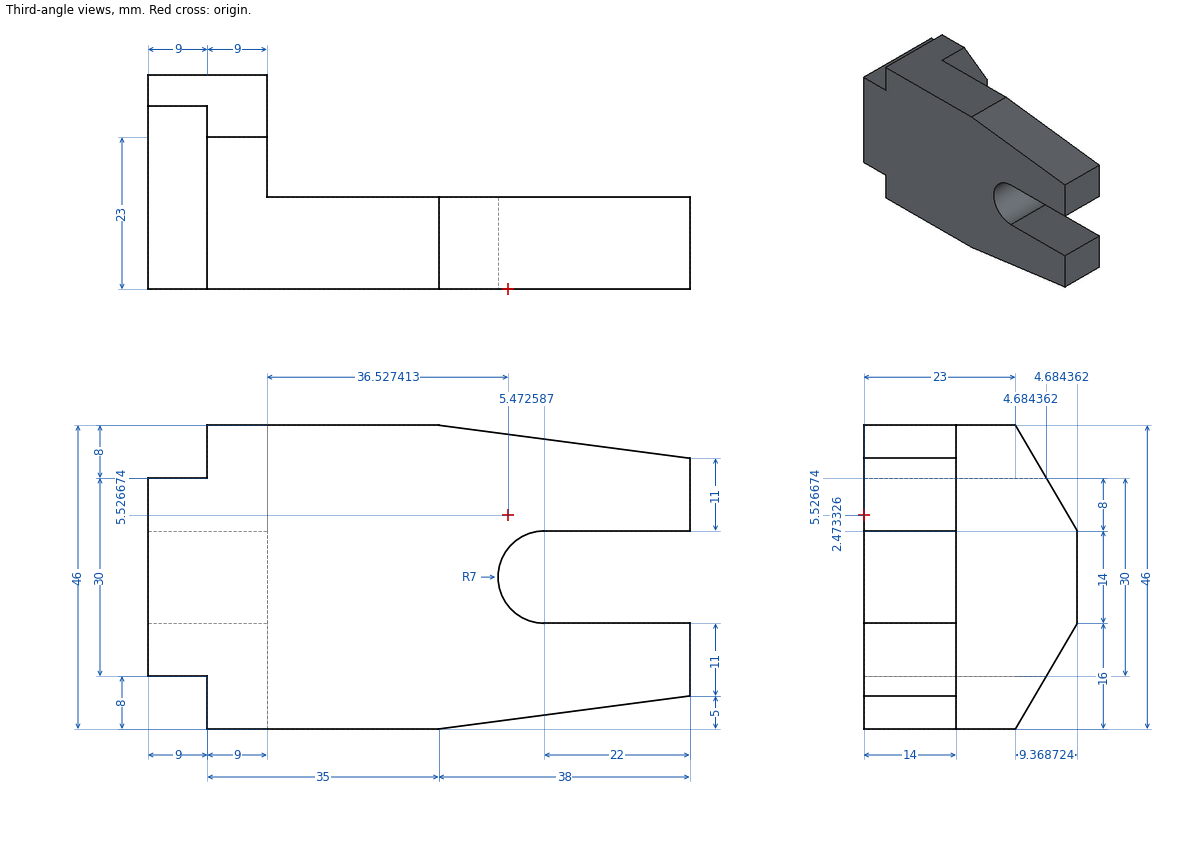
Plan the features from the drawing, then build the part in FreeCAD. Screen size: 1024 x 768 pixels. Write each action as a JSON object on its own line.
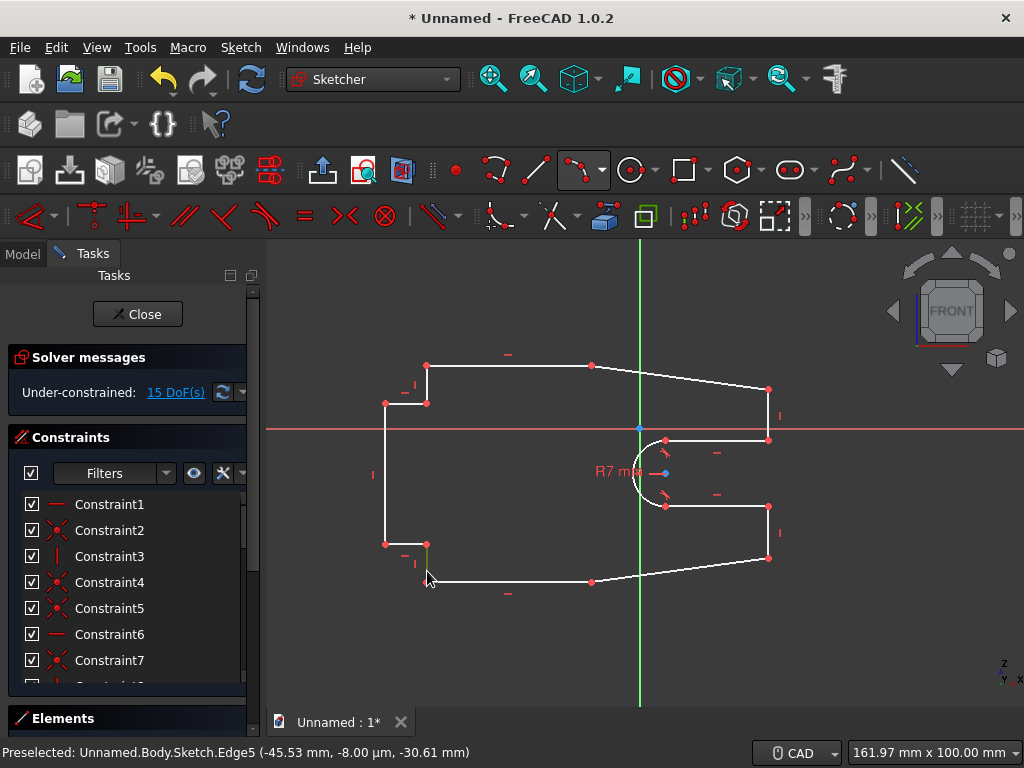
{"action": "left_click", "coordinate": [56, 216]}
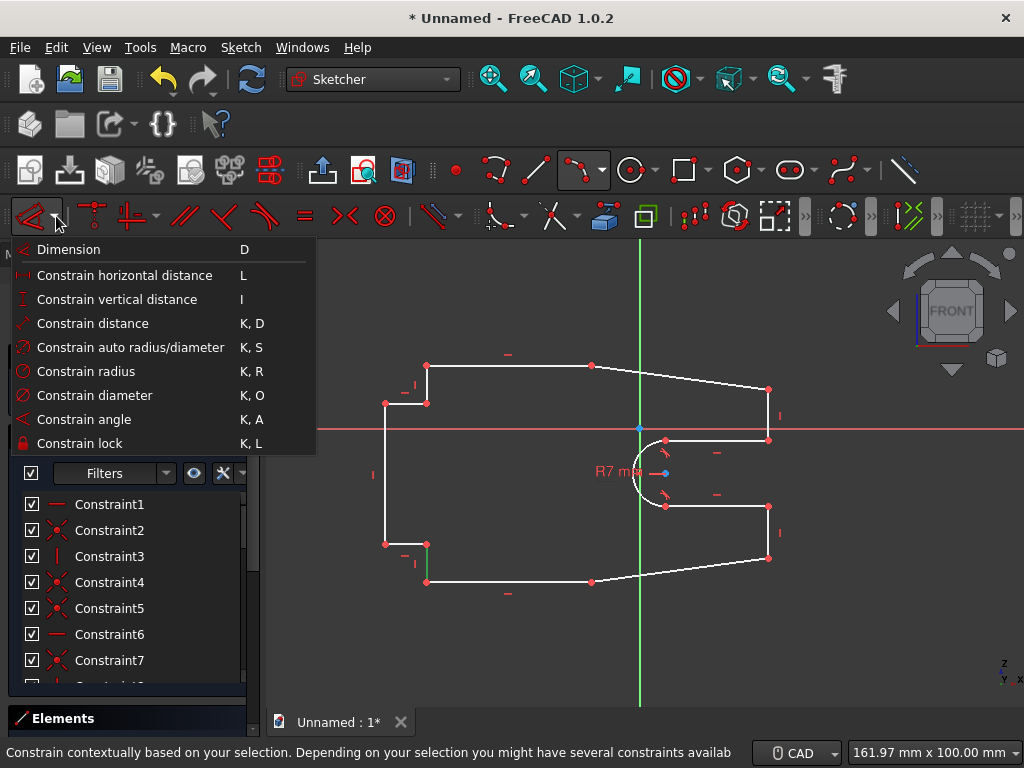
{"action": "left_click", "coordinate": [164, 299]}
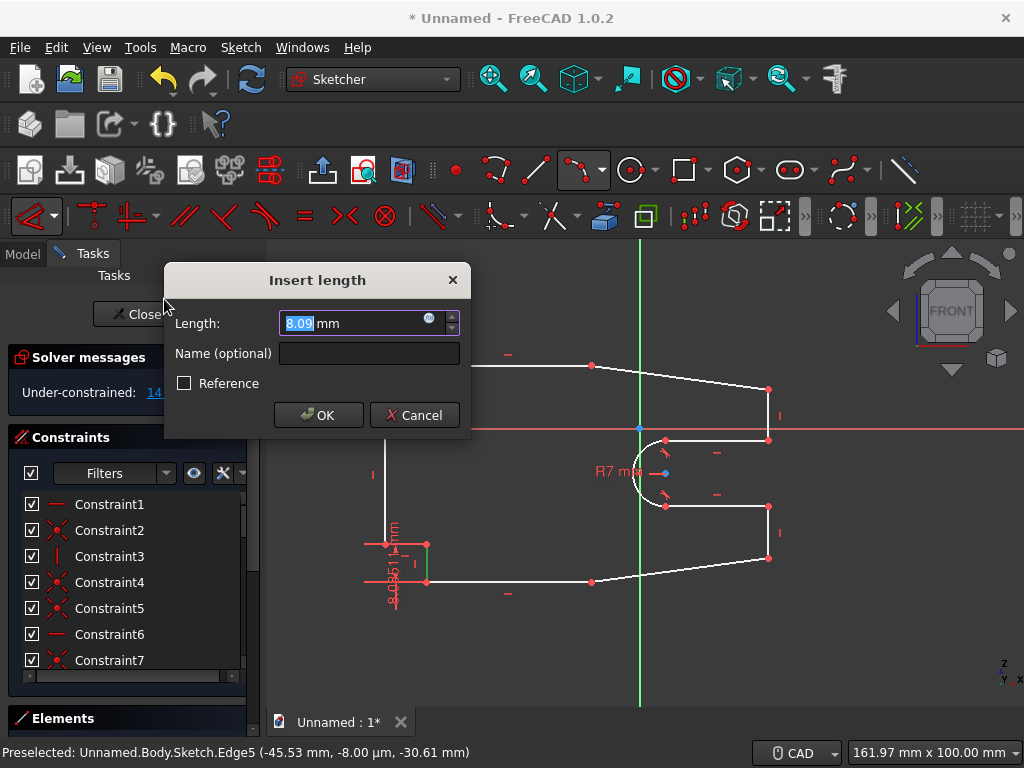
{"action": "type", "text": "8"}
{"action": "key", "text": "Return"}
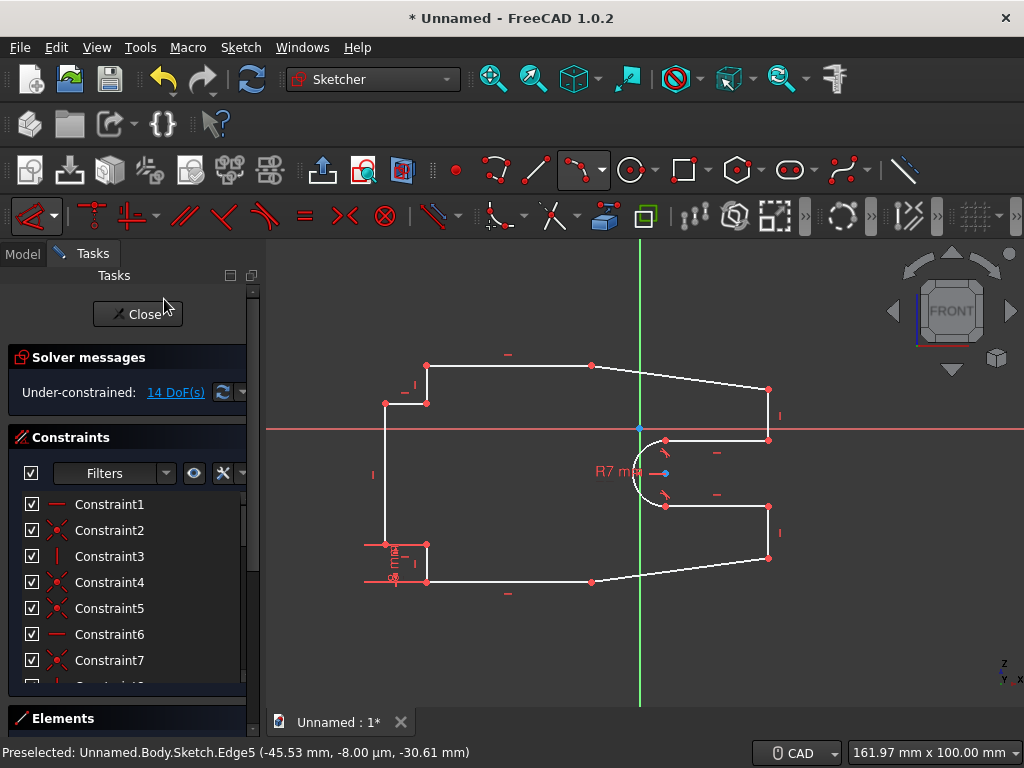
{"action": "left_click", "coordinate": [414, 545]}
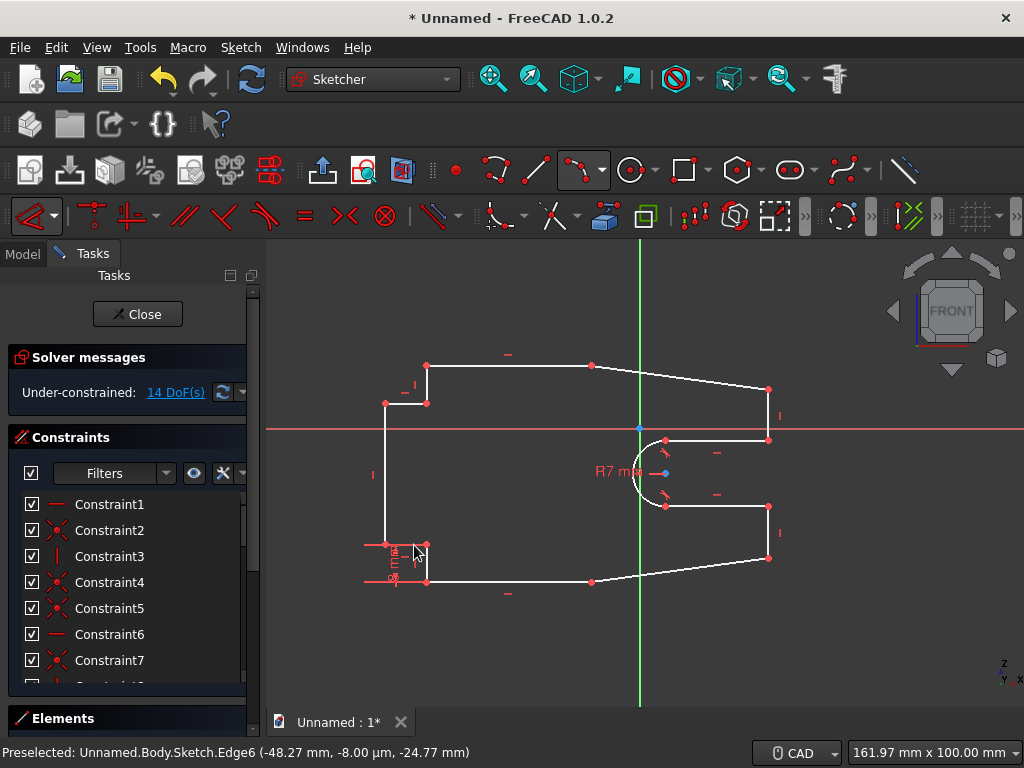
{"action": "left_click", "coordinate": [56, 216]}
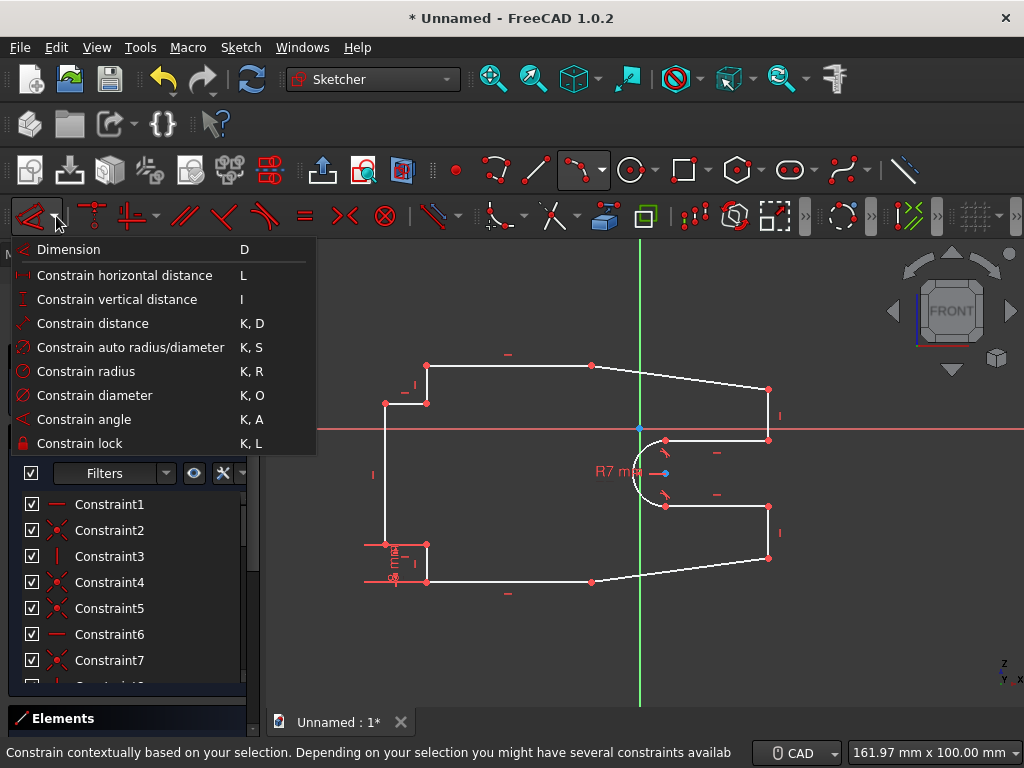
{"action": "left_click", "coordinate": [164, 275]}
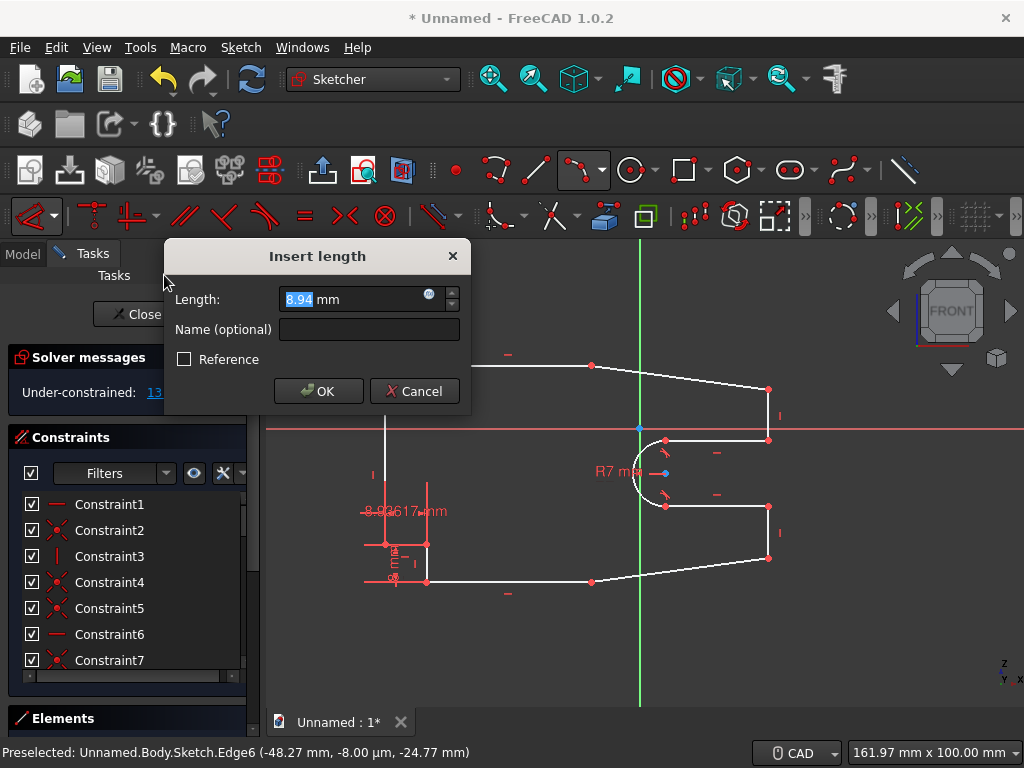
{"action": "type", "text": "9"}
{"action": "key", "text": "Return"}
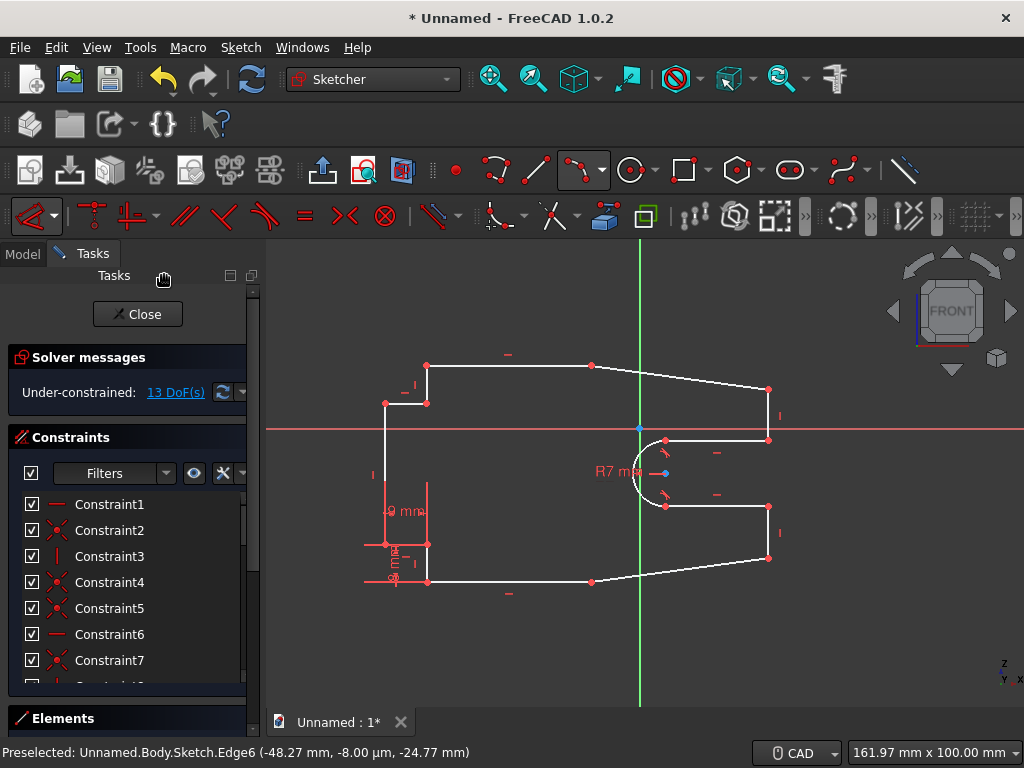
{"action": "left_click", "coordinate": [398, 404]}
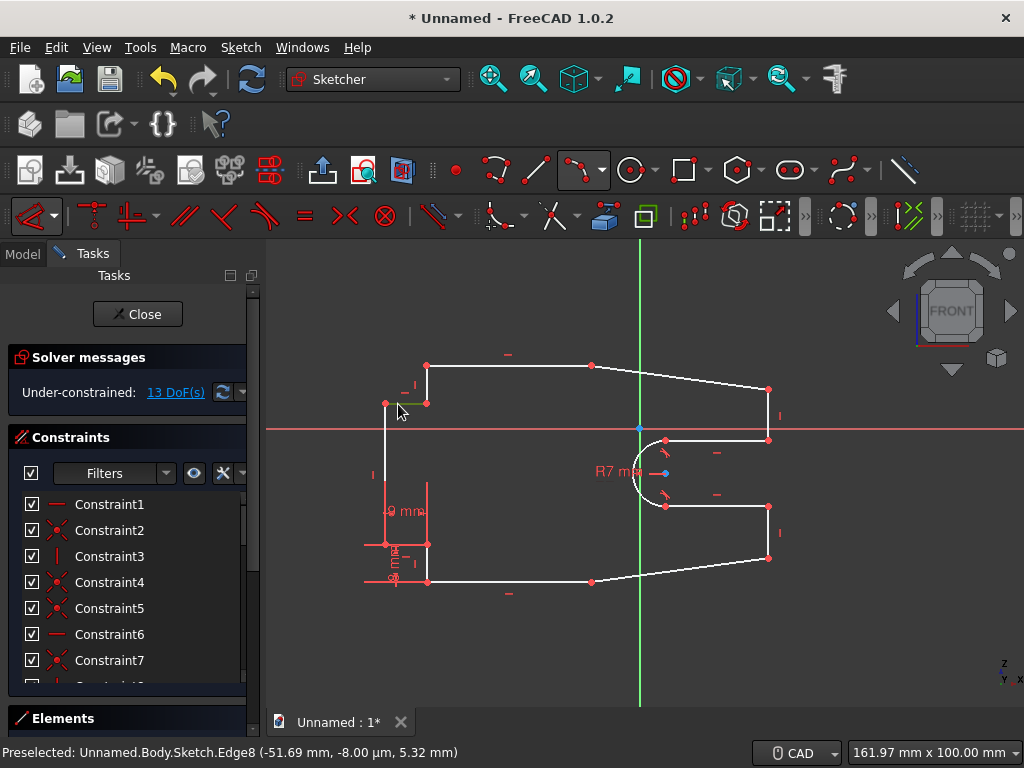
{"action": "key", "text": "l"}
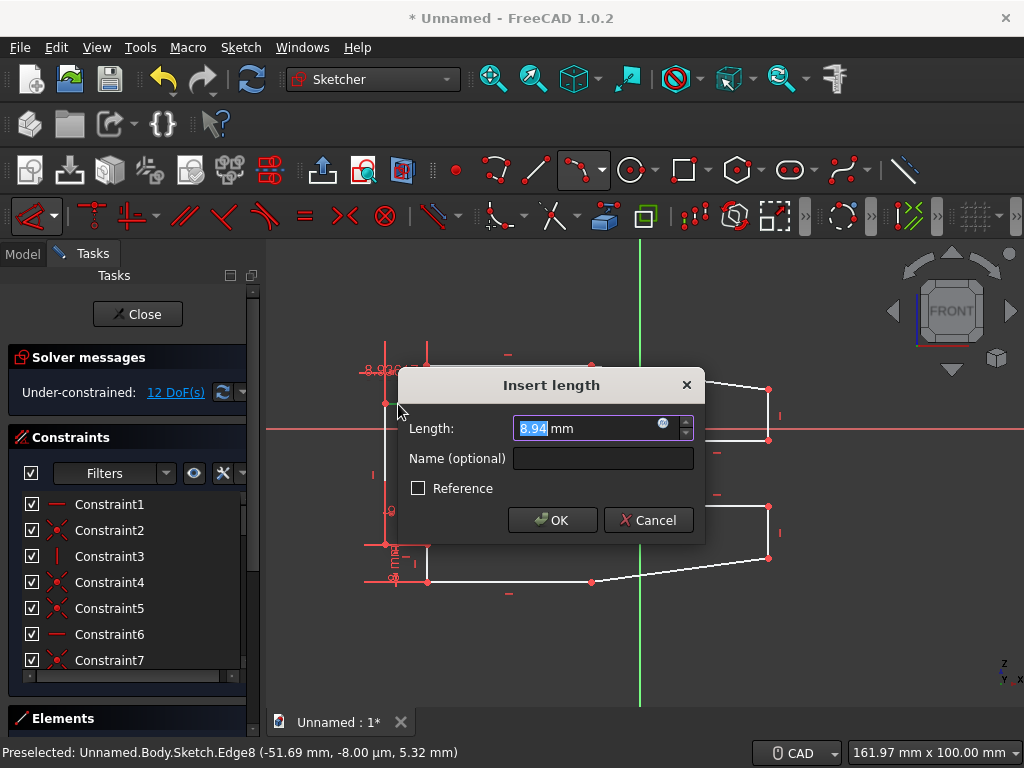
{"action": "type", "text": "9"}
{"action": "key", "text": "Return"}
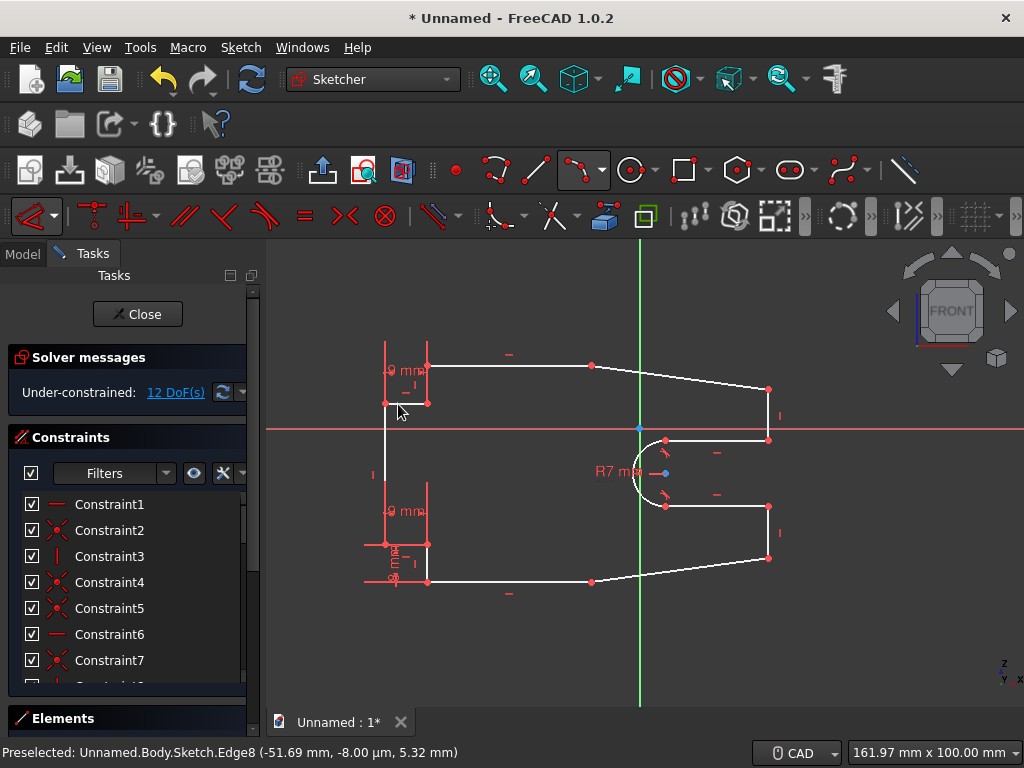
{"action": "left_click", "coordinate": [427, 392]}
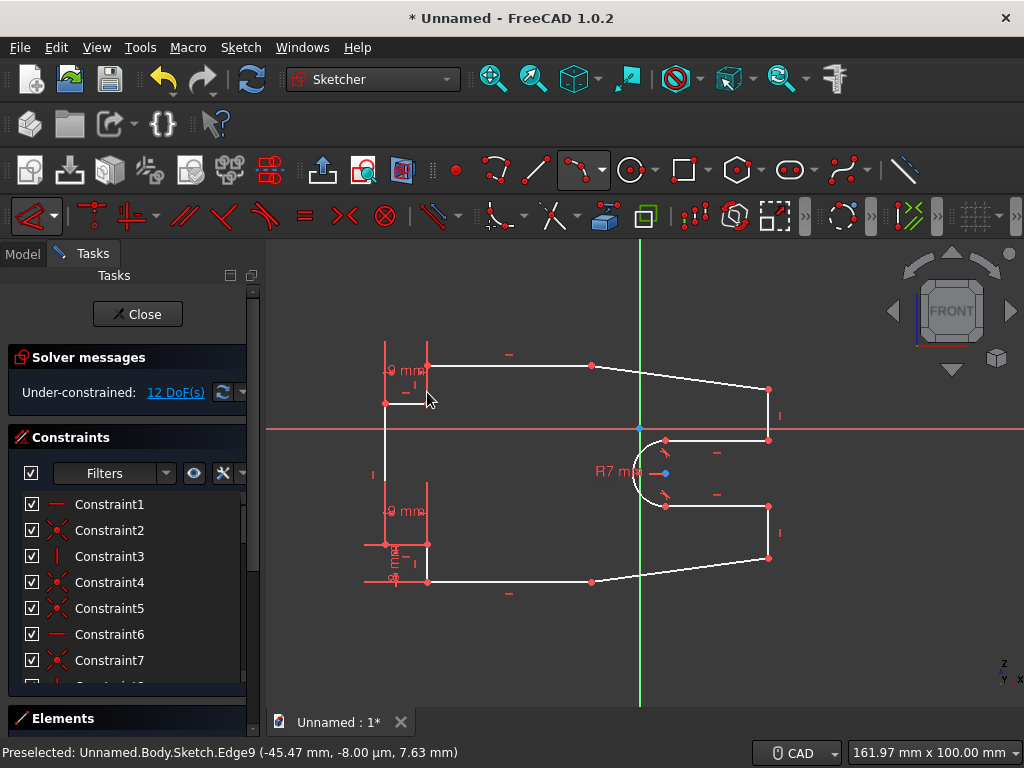
{"action": "key", "text": "i"}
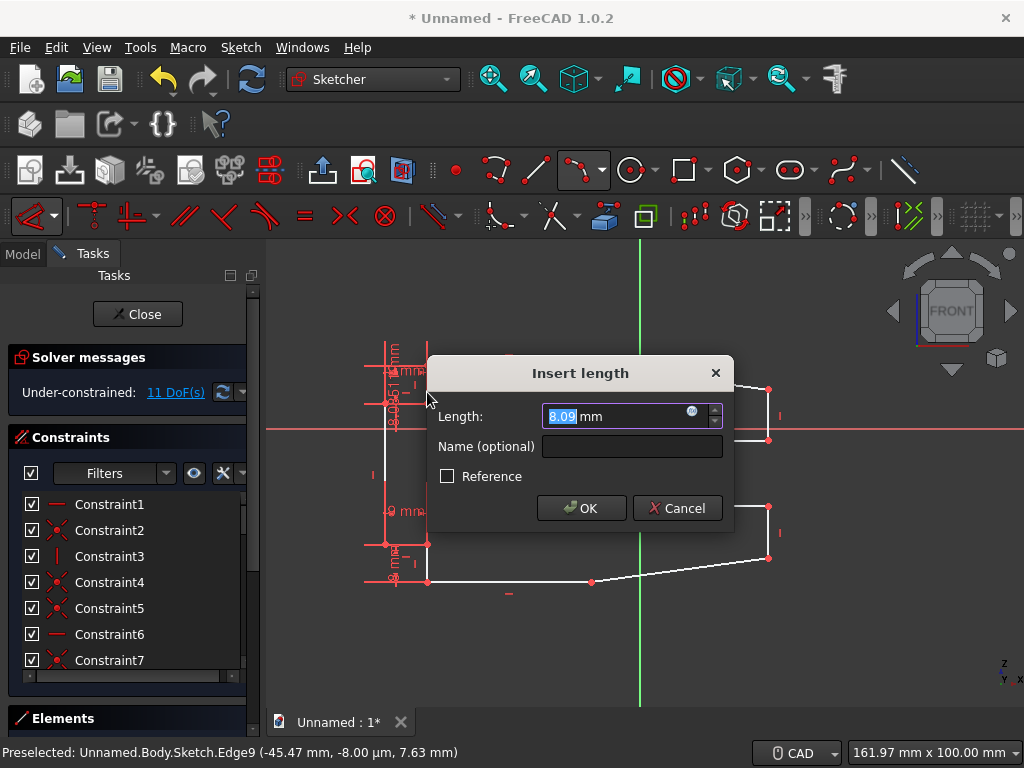
{"action": "type", "text": "8"}
{"action": "key", "text": "Return"}